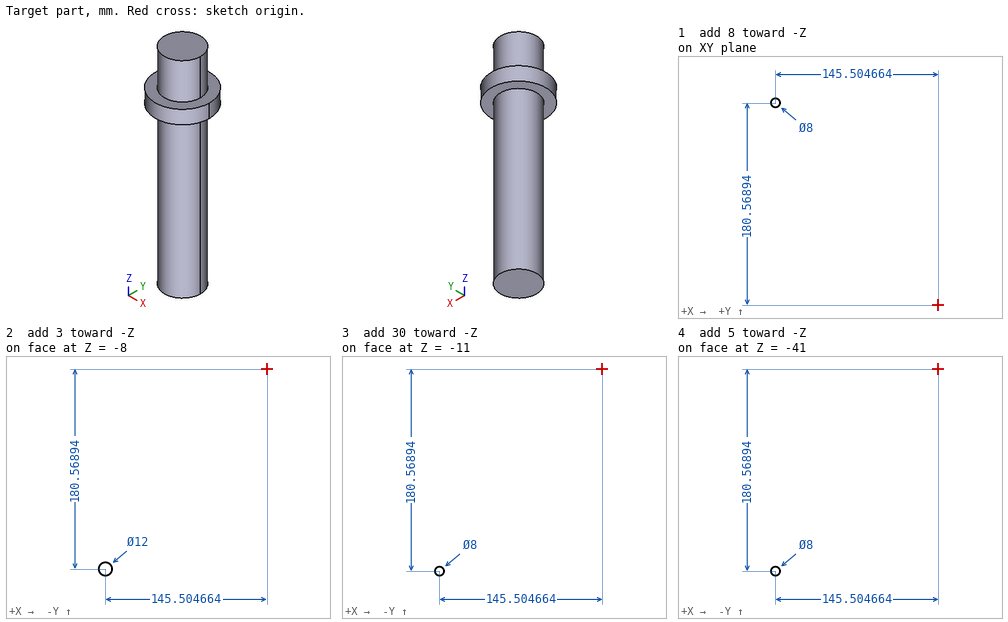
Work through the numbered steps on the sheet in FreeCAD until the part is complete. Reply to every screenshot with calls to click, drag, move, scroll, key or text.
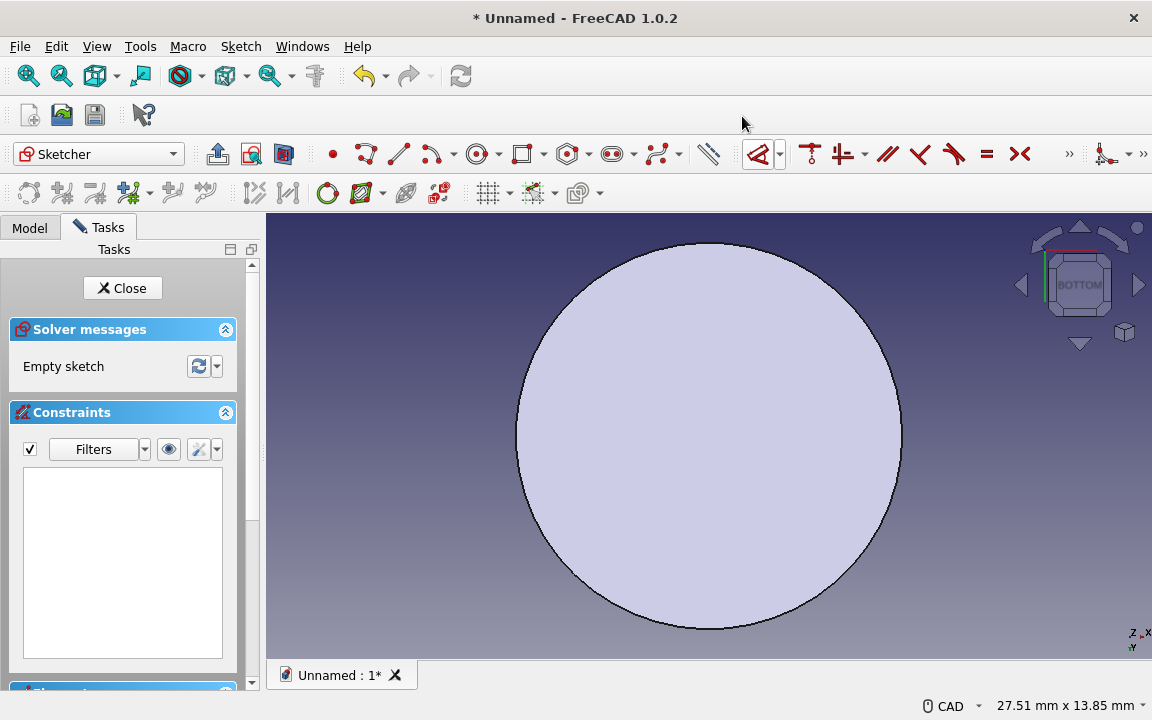
click(476, 154)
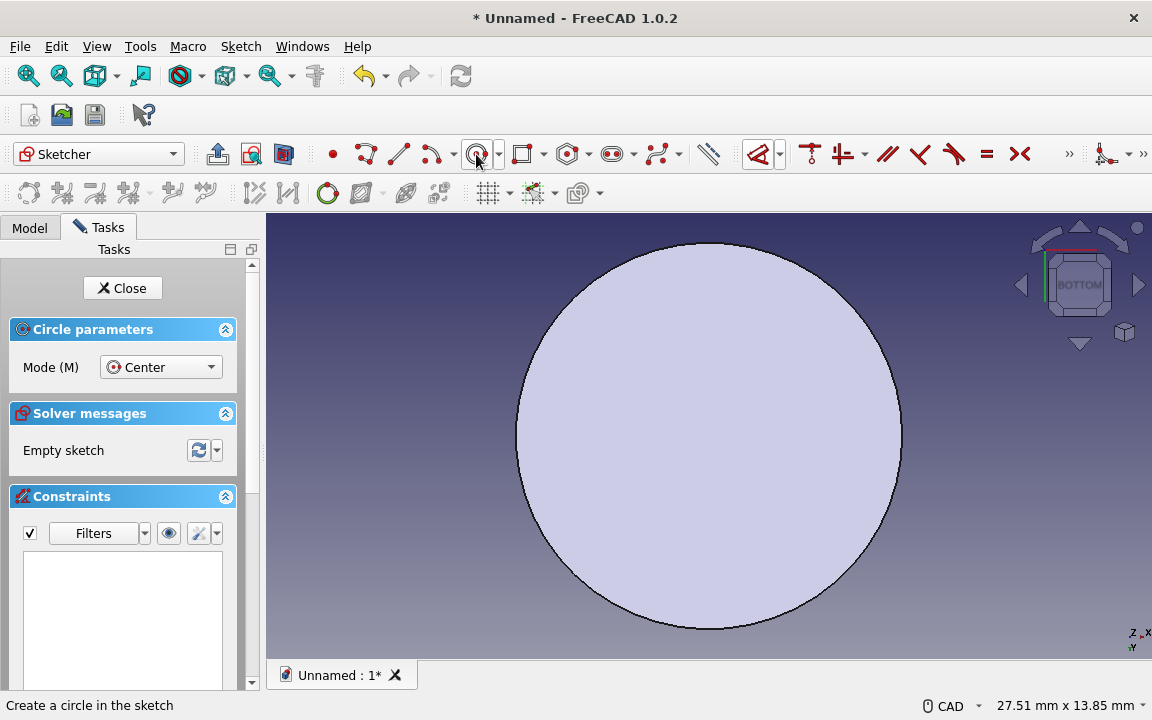
click(709, 436)
click(800, 345)
key(Escape)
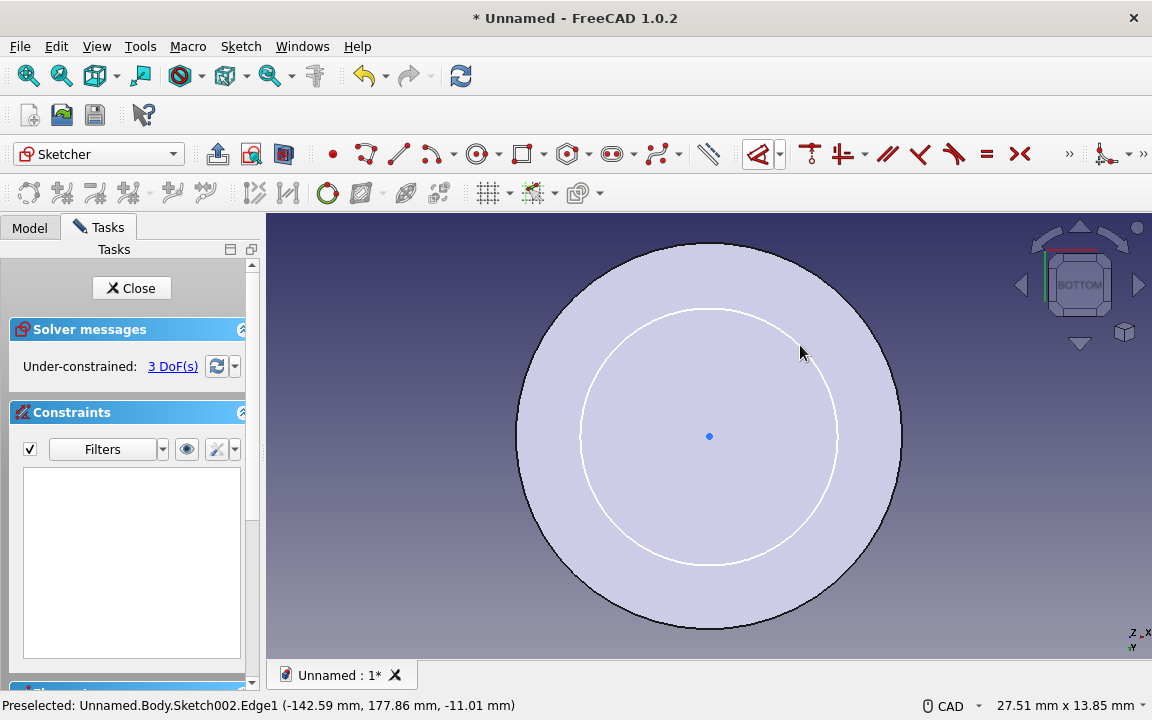
click(800, 346)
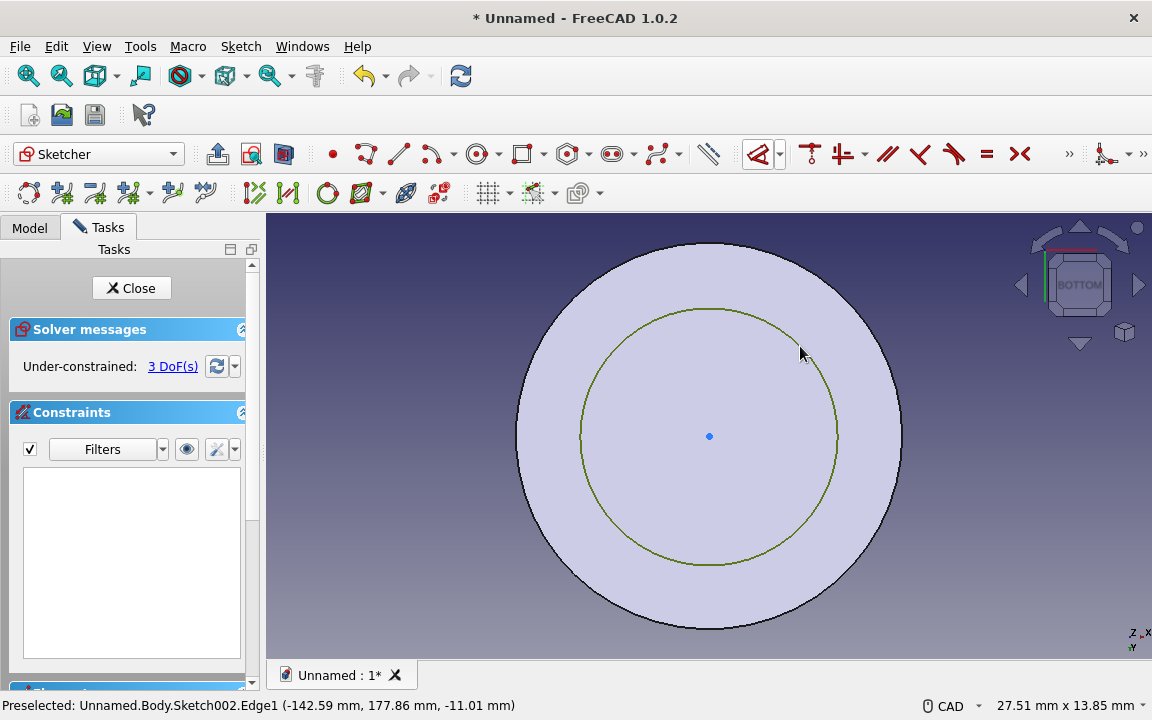
key(k)
key(o)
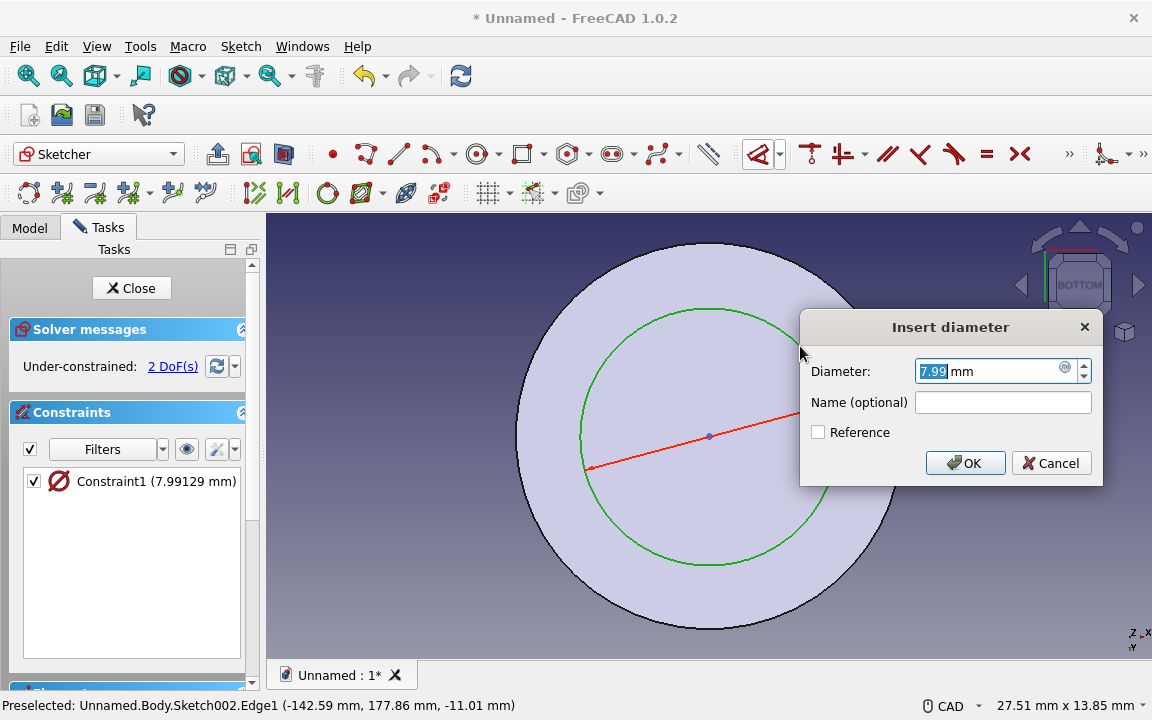
text(8)
key(Return)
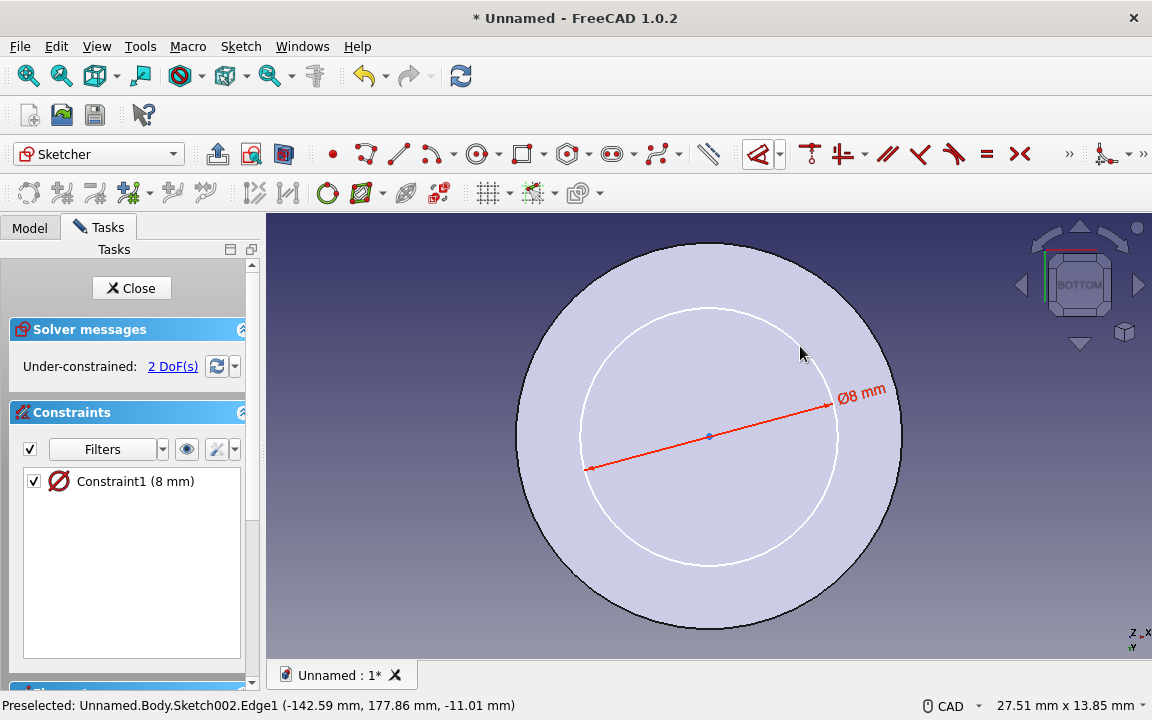
click(709, 437)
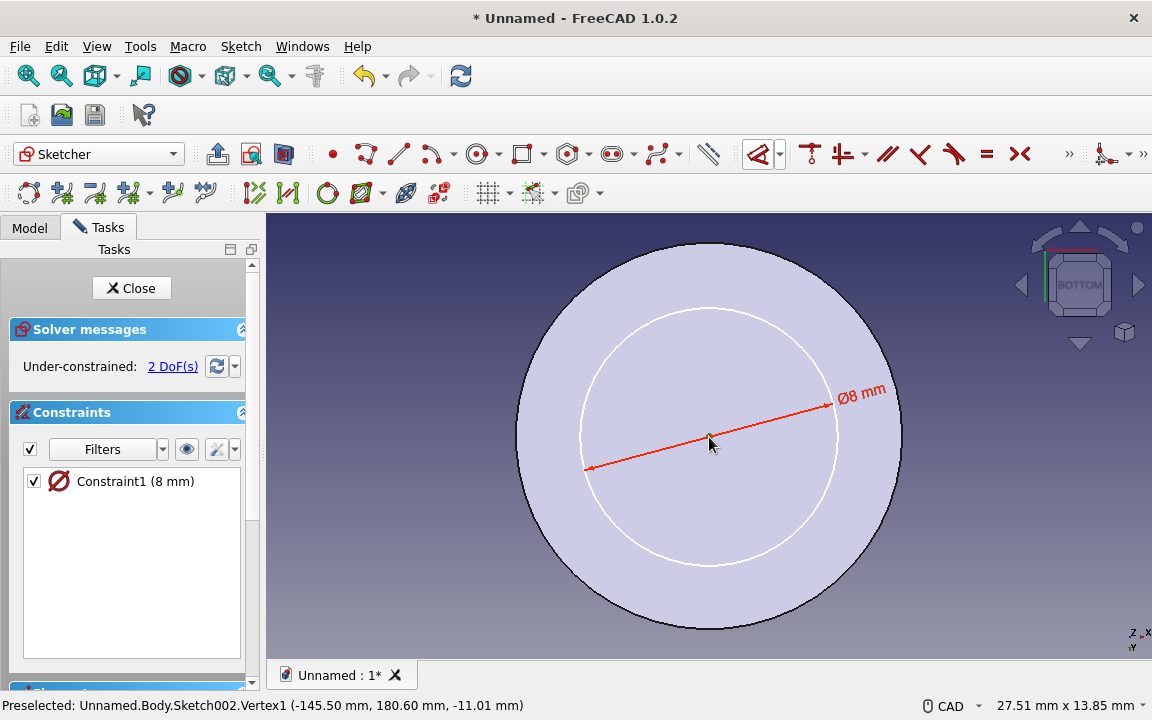
click(780, 154)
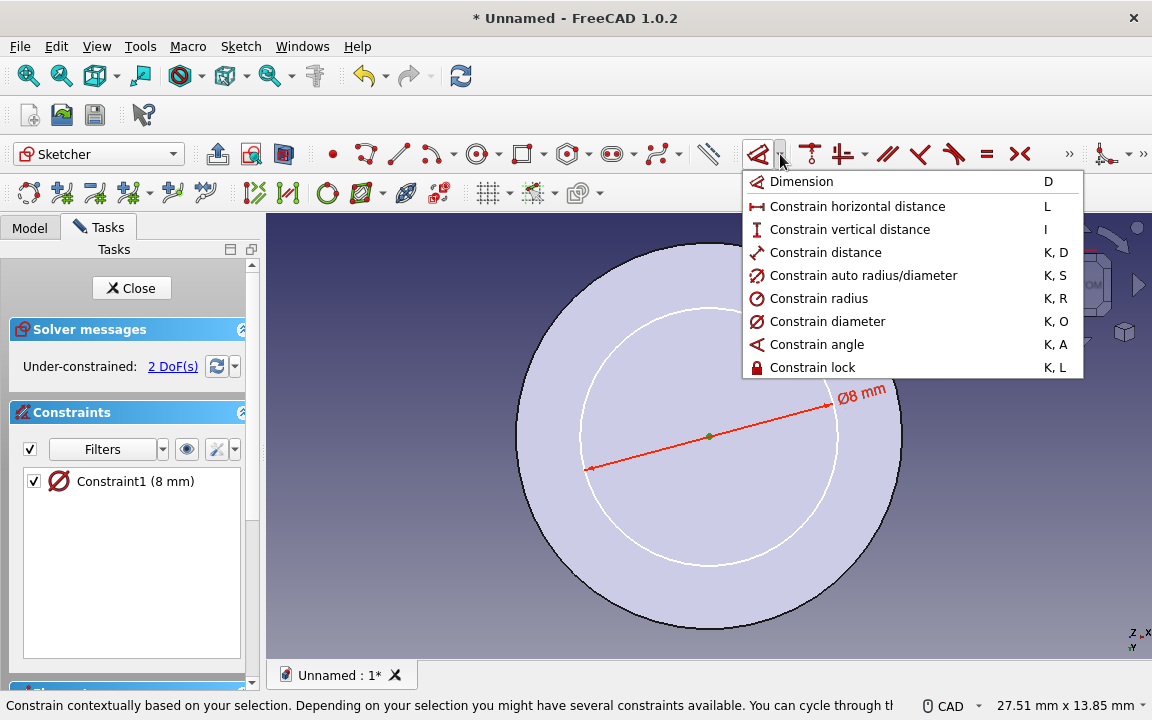
click(913, 230)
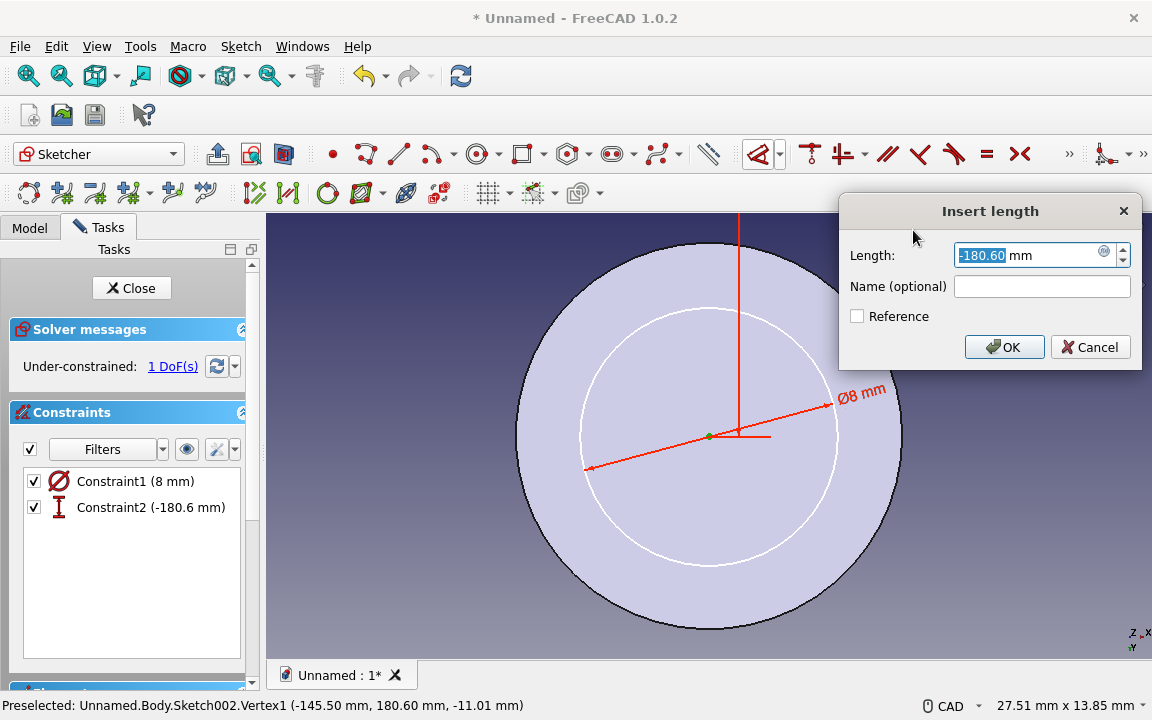
text(-180.56894)
key(Return)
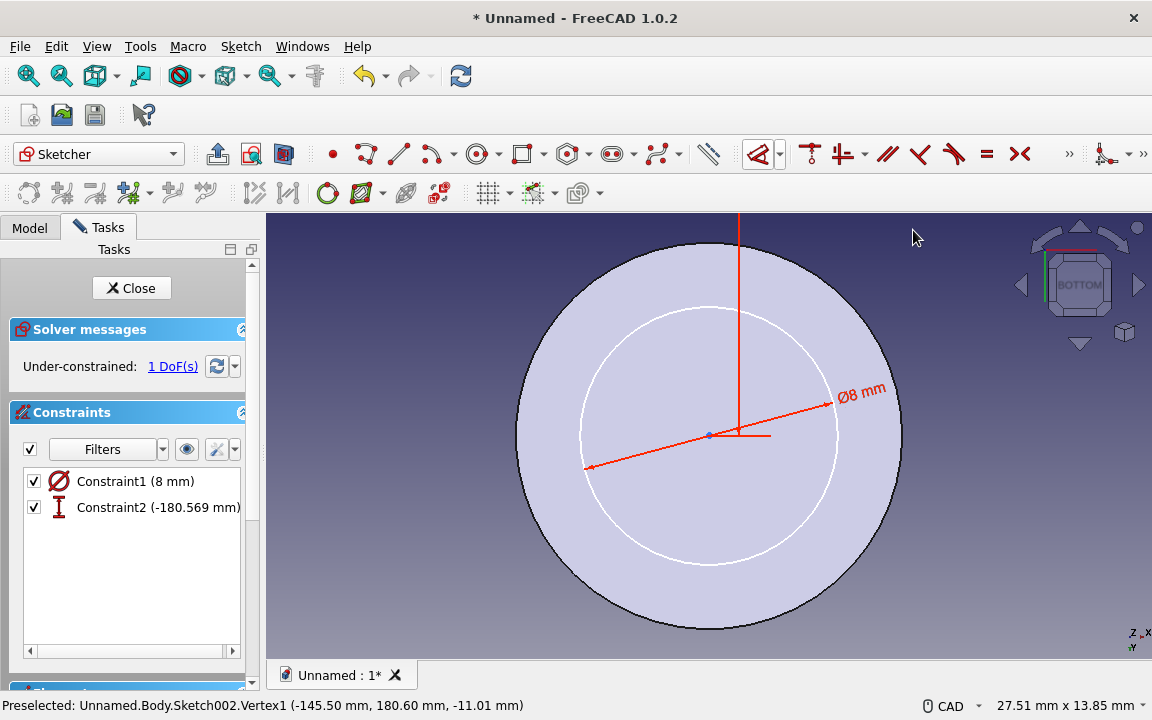
click(709, 436)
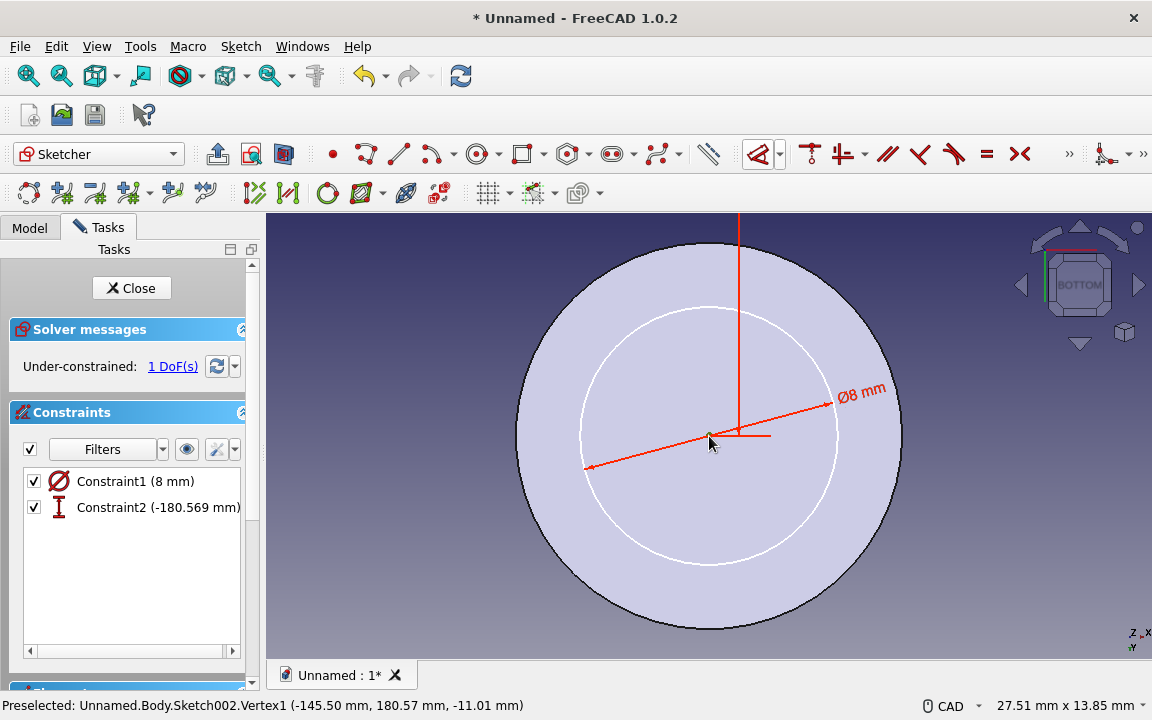
click(780, 154)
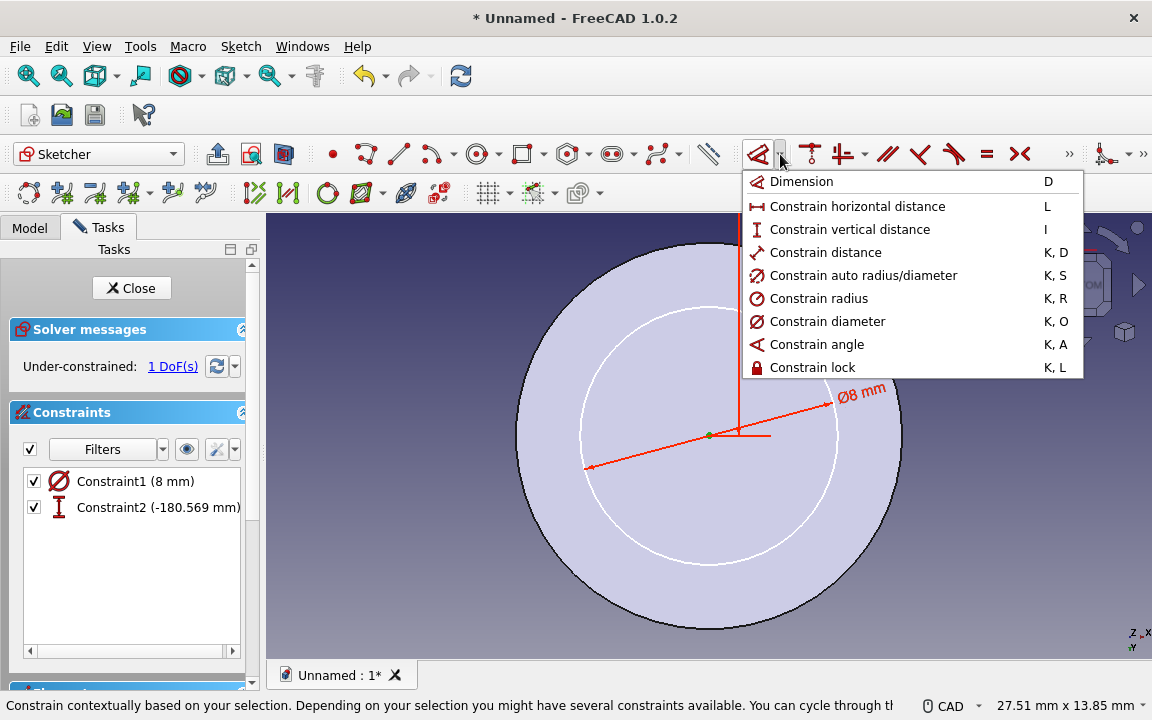
click(913, 206)